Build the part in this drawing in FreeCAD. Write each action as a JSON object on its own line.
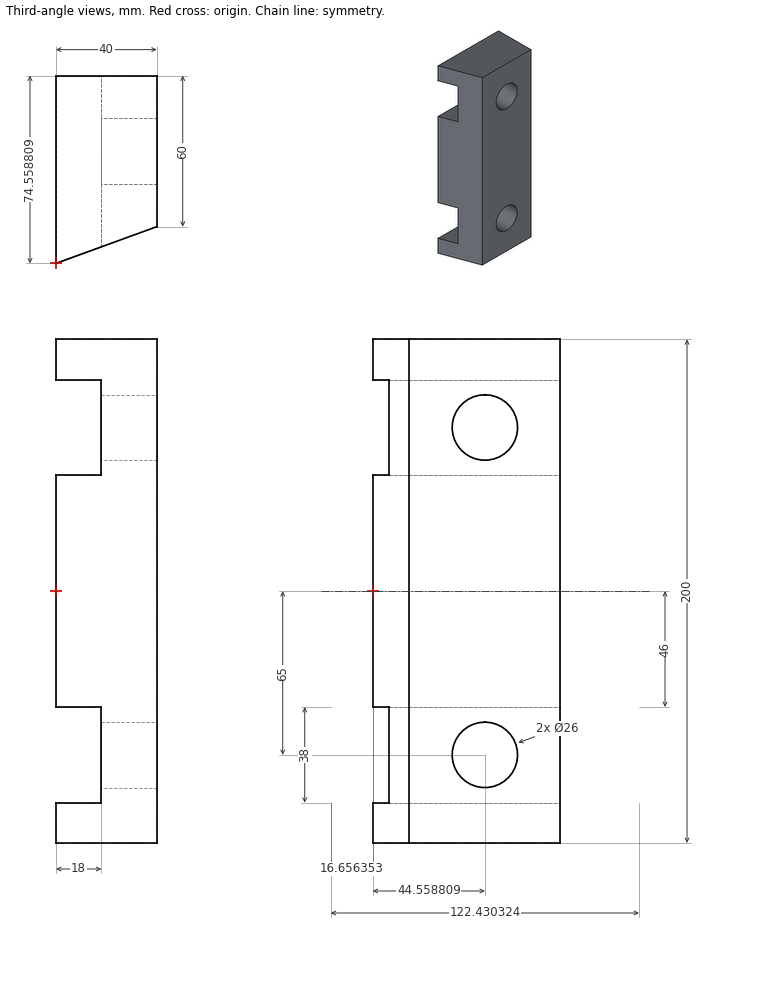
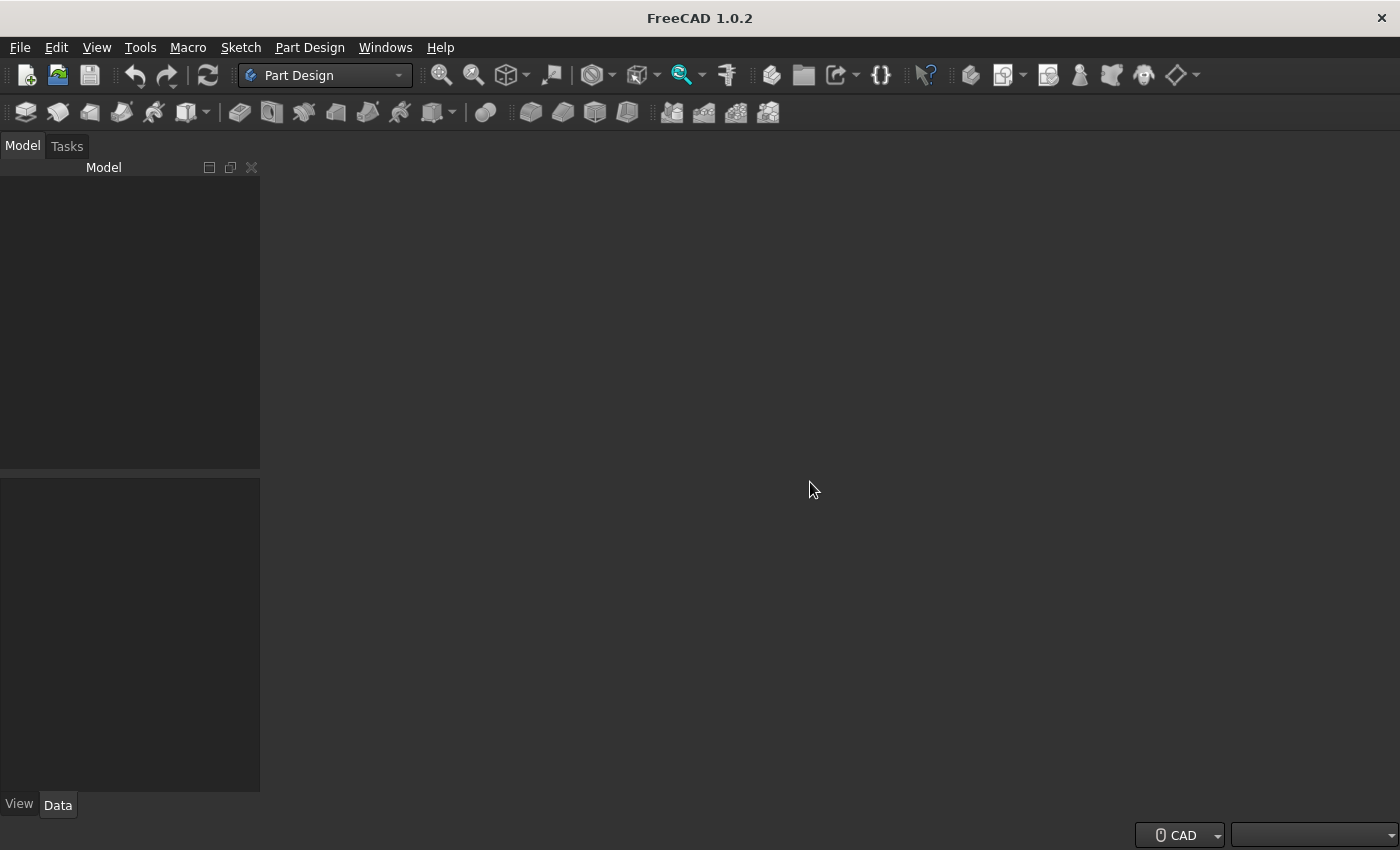
{"action": "left_click", "coordinate": [26, 76]}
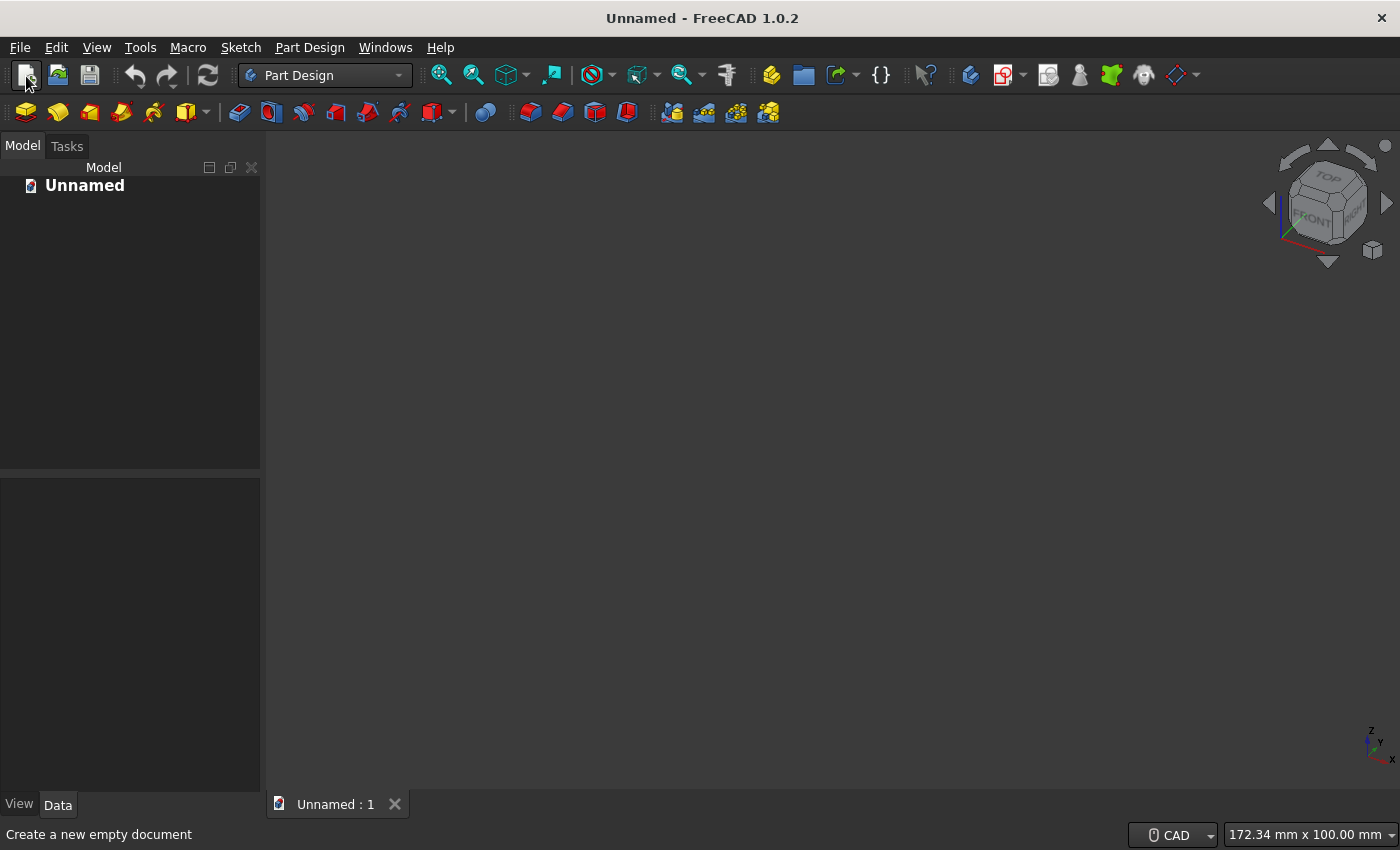
{"action": "left_click", "coordinate": [1004, 76]}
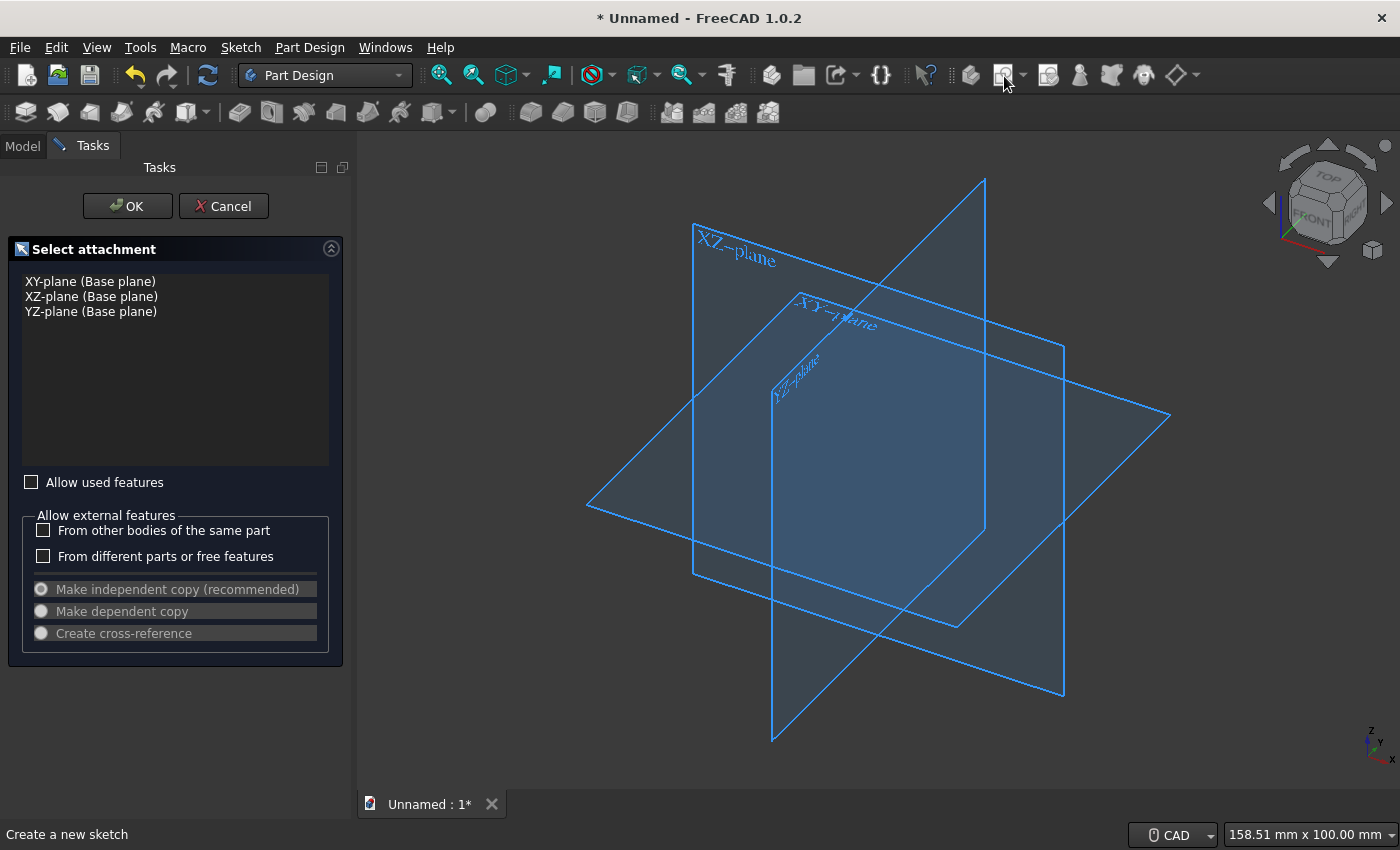
{"action": "left_click", "coordinate": [82, 282]}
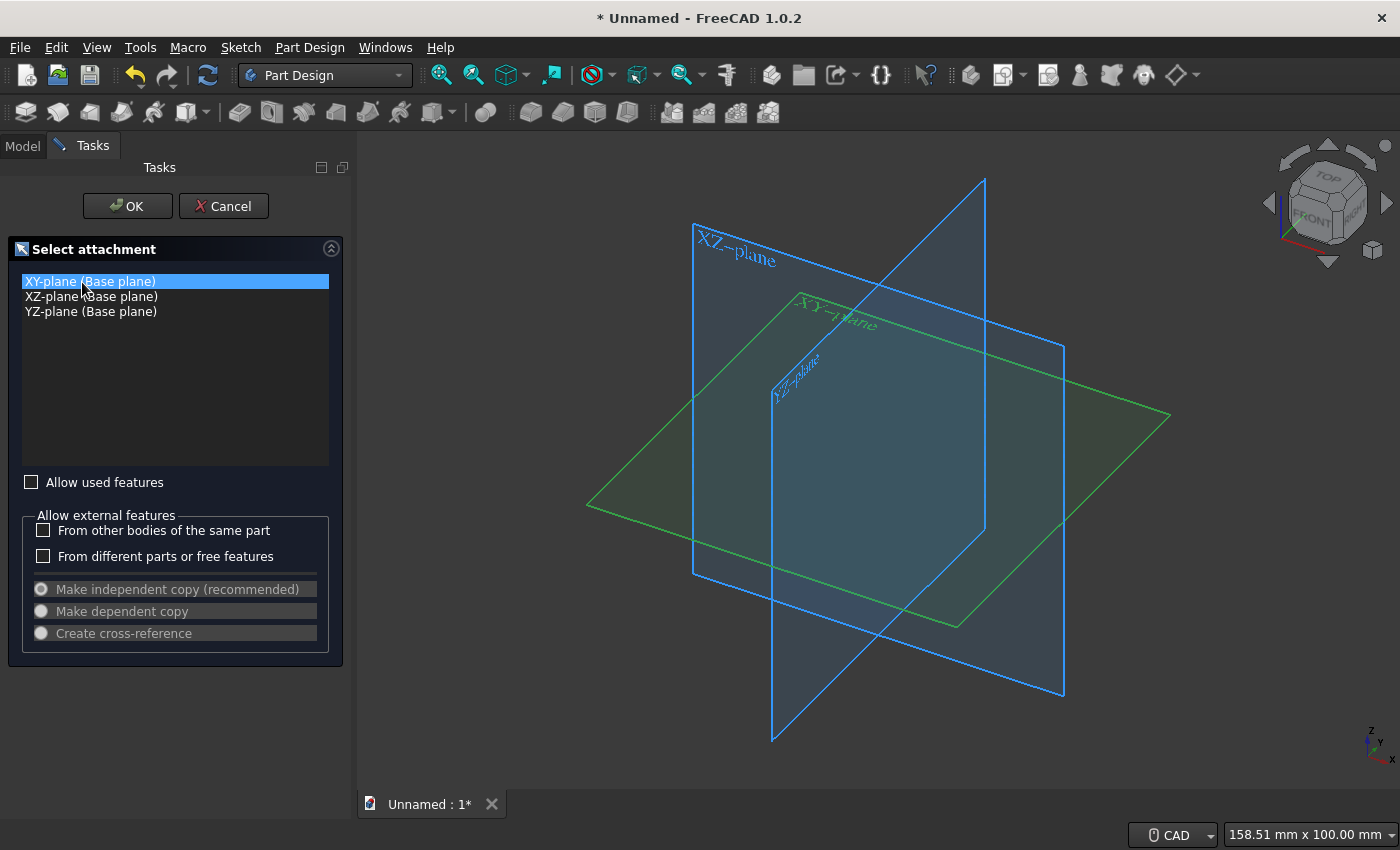
{"action": "left_click", "coordinate": [128, 206]}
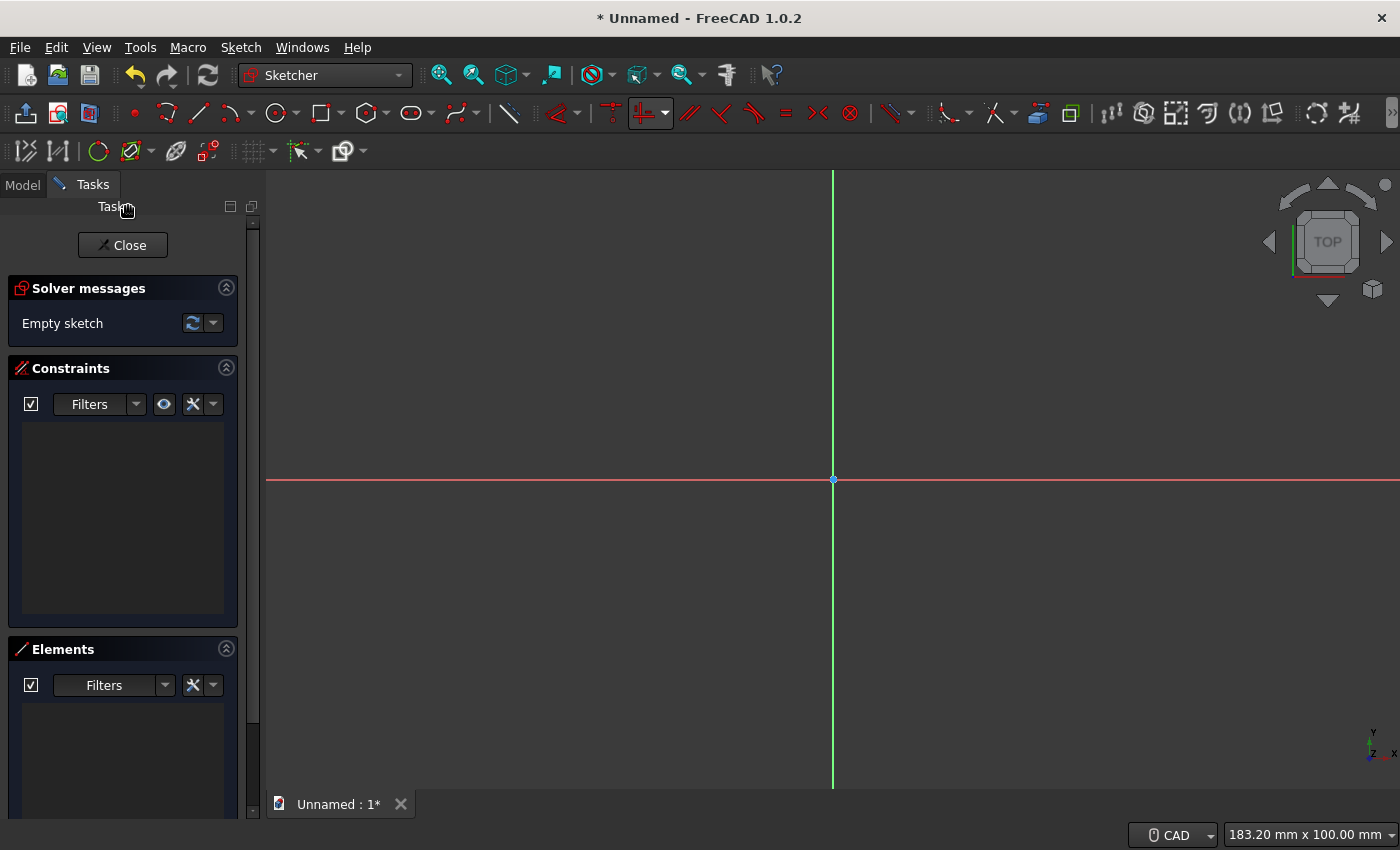
{"action": "scroll", "coordinate": [374, 761], "scroll_direction": "down", "scroll_amount": 2}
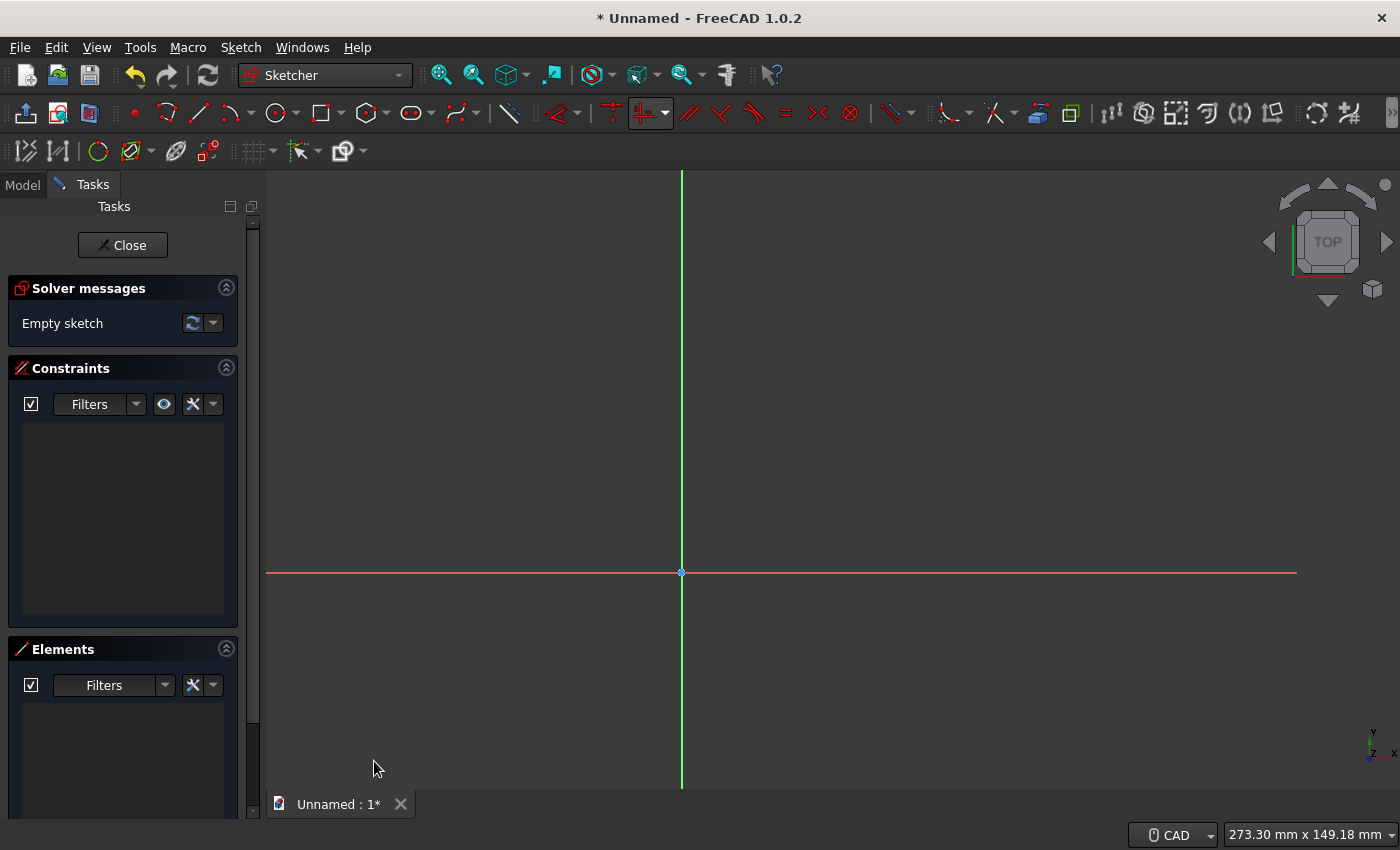
{"action": "left_click", "coordinate": [168, 114]}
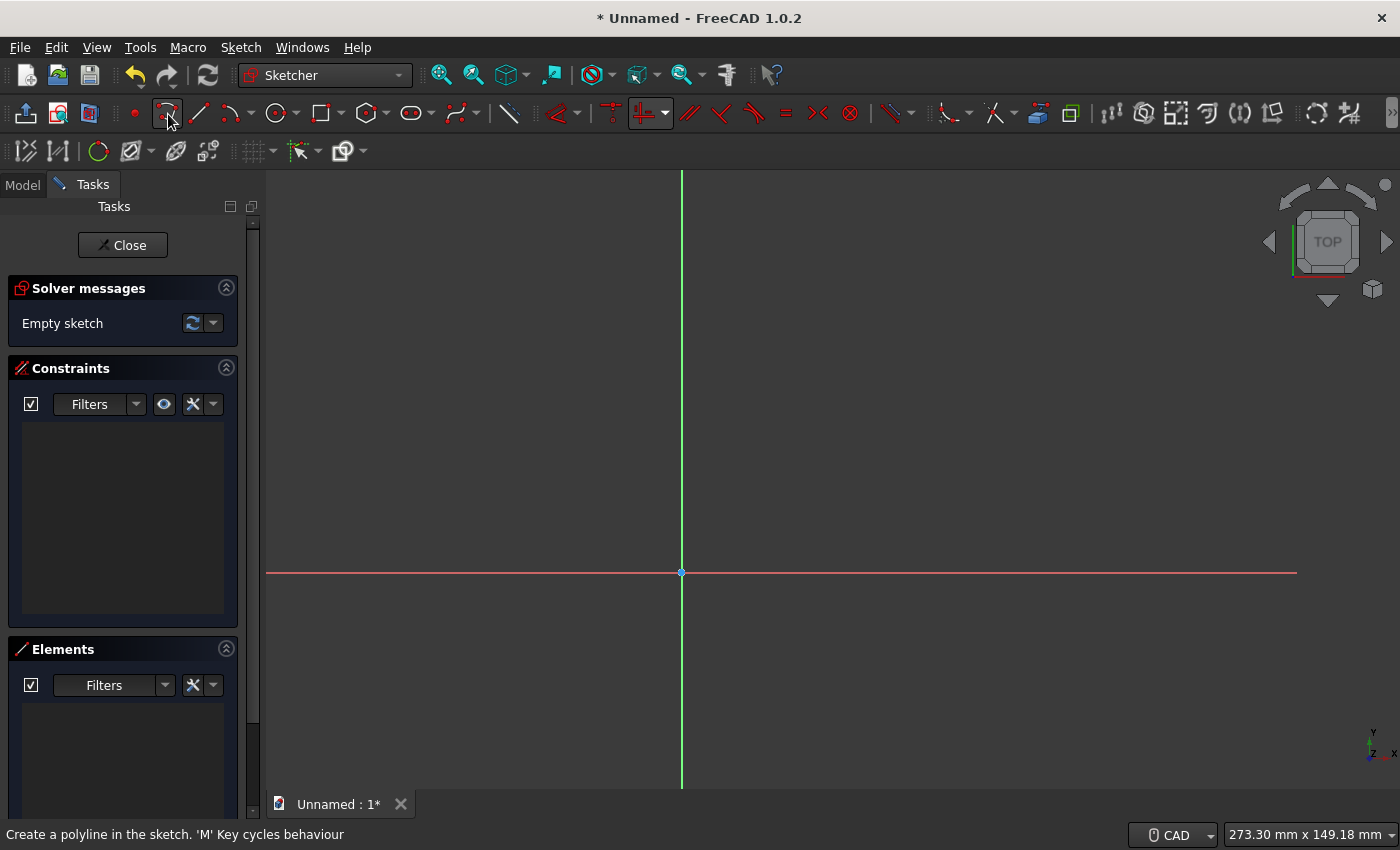
{"action": "left_click", "coordinate": [682, 573]}
{"action": "left_click", "coordinate": [848, 512]}
{"action": "left_click", "coordinate": [848, 263]}
{"action": "left_click", "coordinate": [691, 263]}
{"action": "left_click", "coordinate": [682, 573]}
{"action": "key", "text": "Escape"}
{"action": "key", "text": "Escape"}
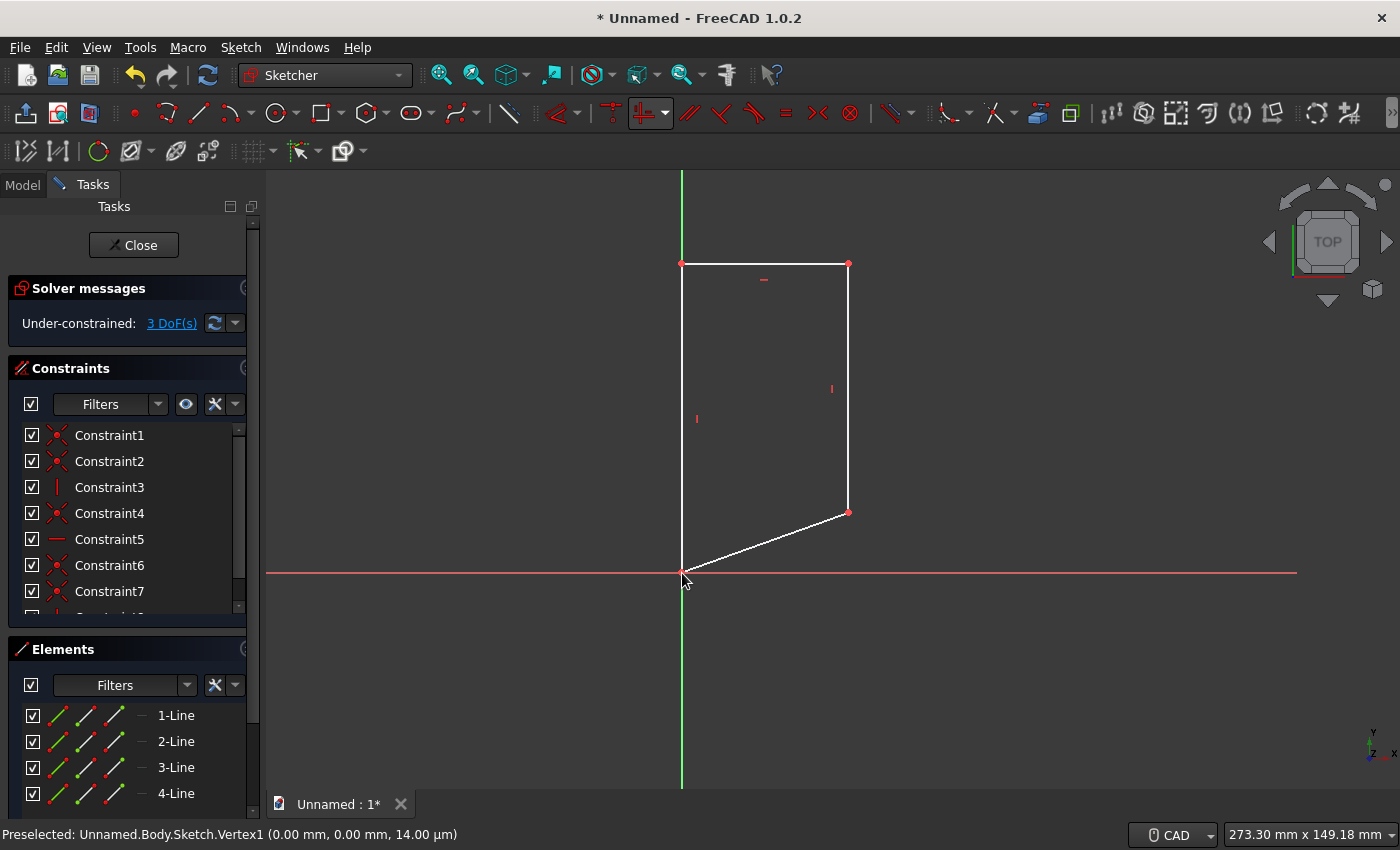
{"action": "left_click", "coordinate": [556, 114]}